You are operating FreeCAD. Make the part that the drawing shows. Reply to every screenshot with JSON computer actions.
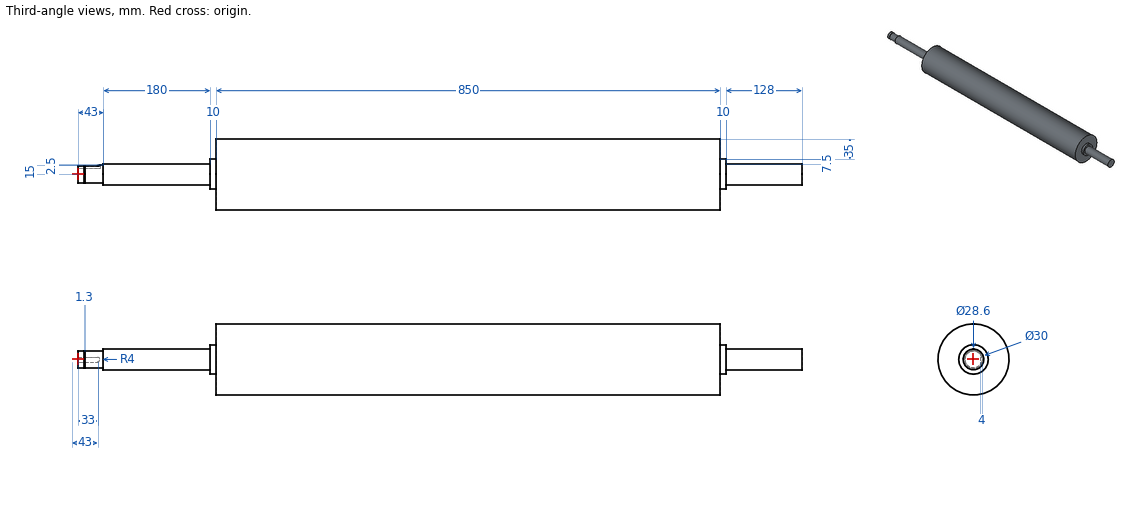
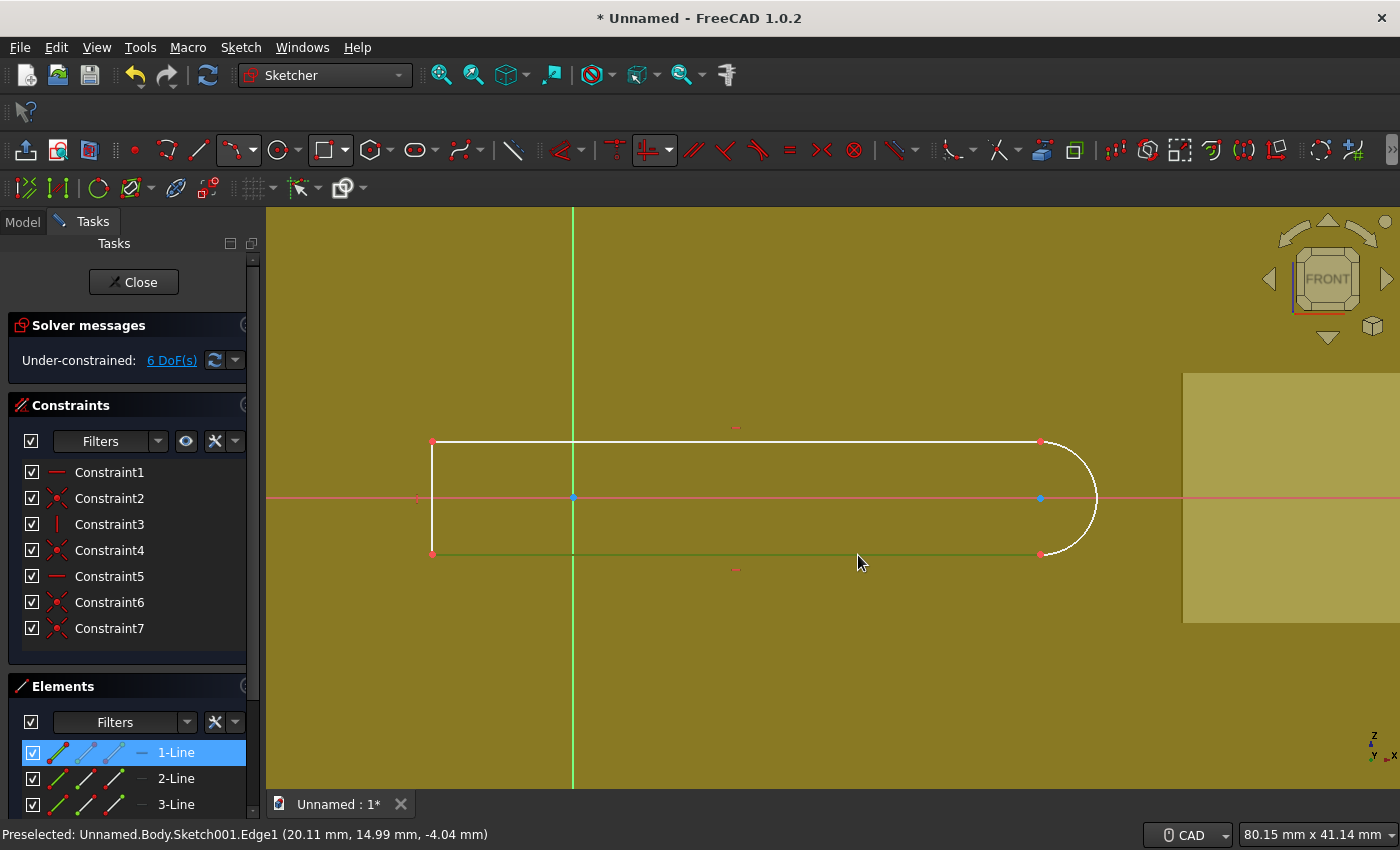
{"action": "left_click", "coordinate": [1086, 532]}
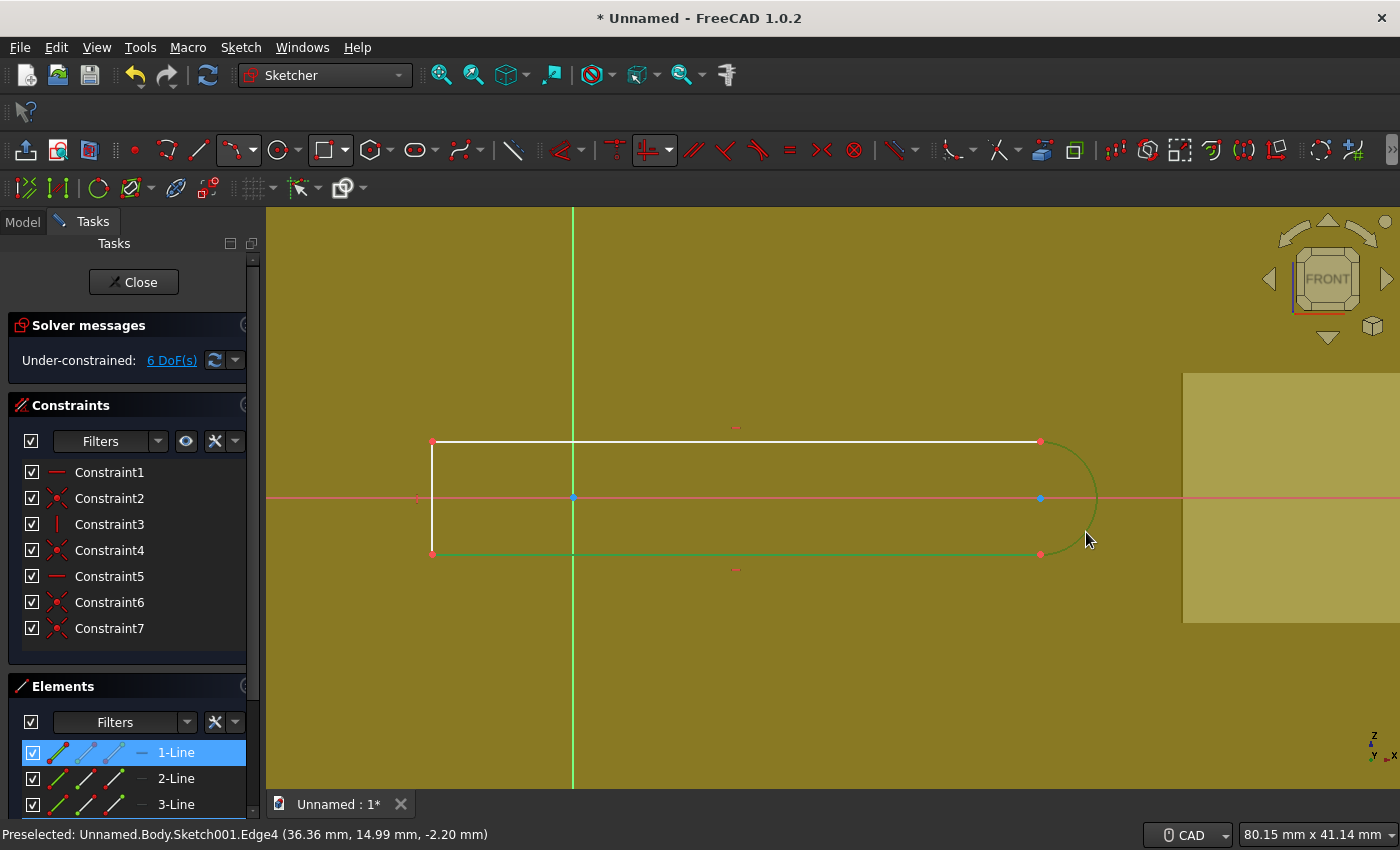
{"action": "key", "text": "t"}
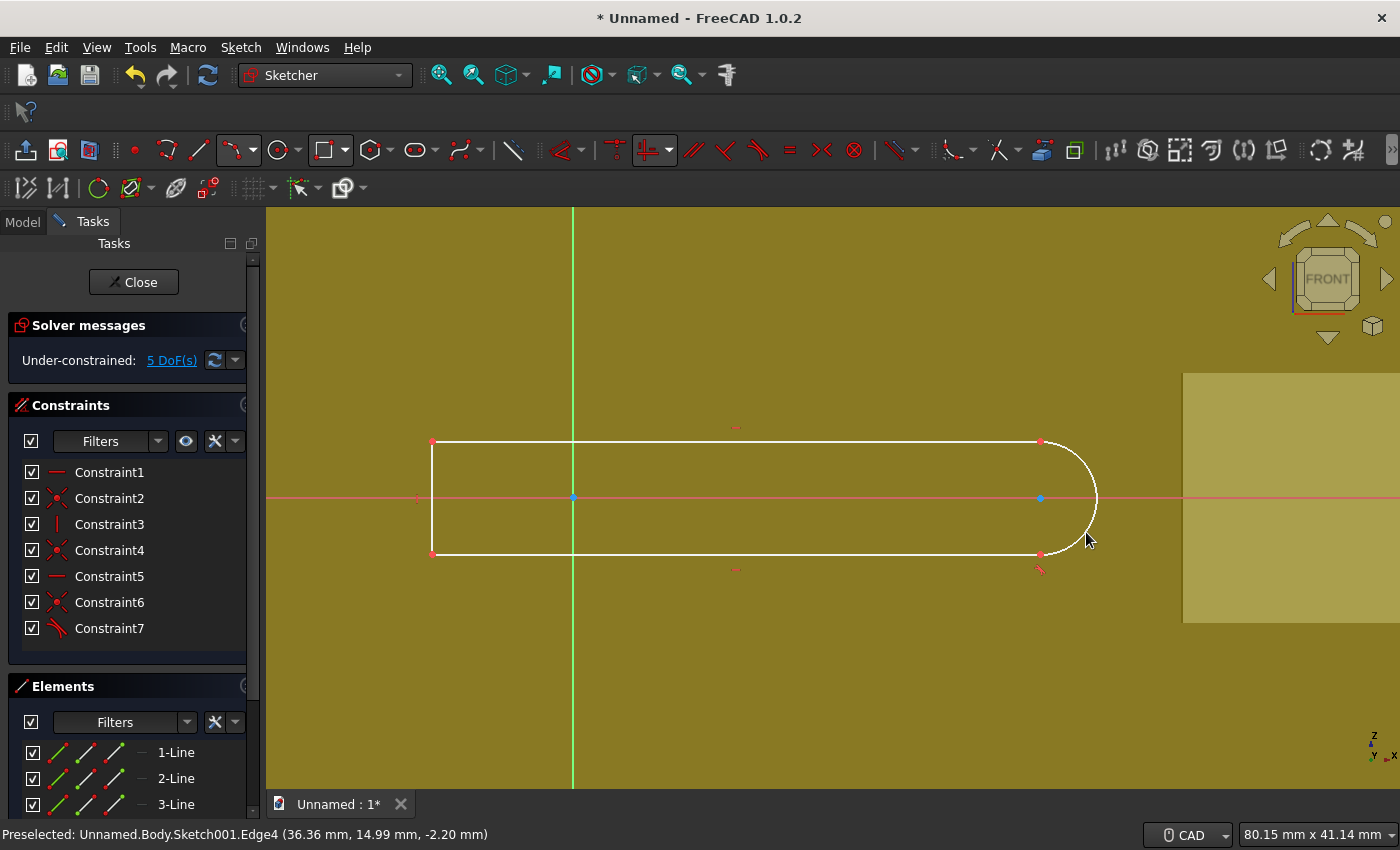
{"action": "left_click", "coordinate": [614, 442]}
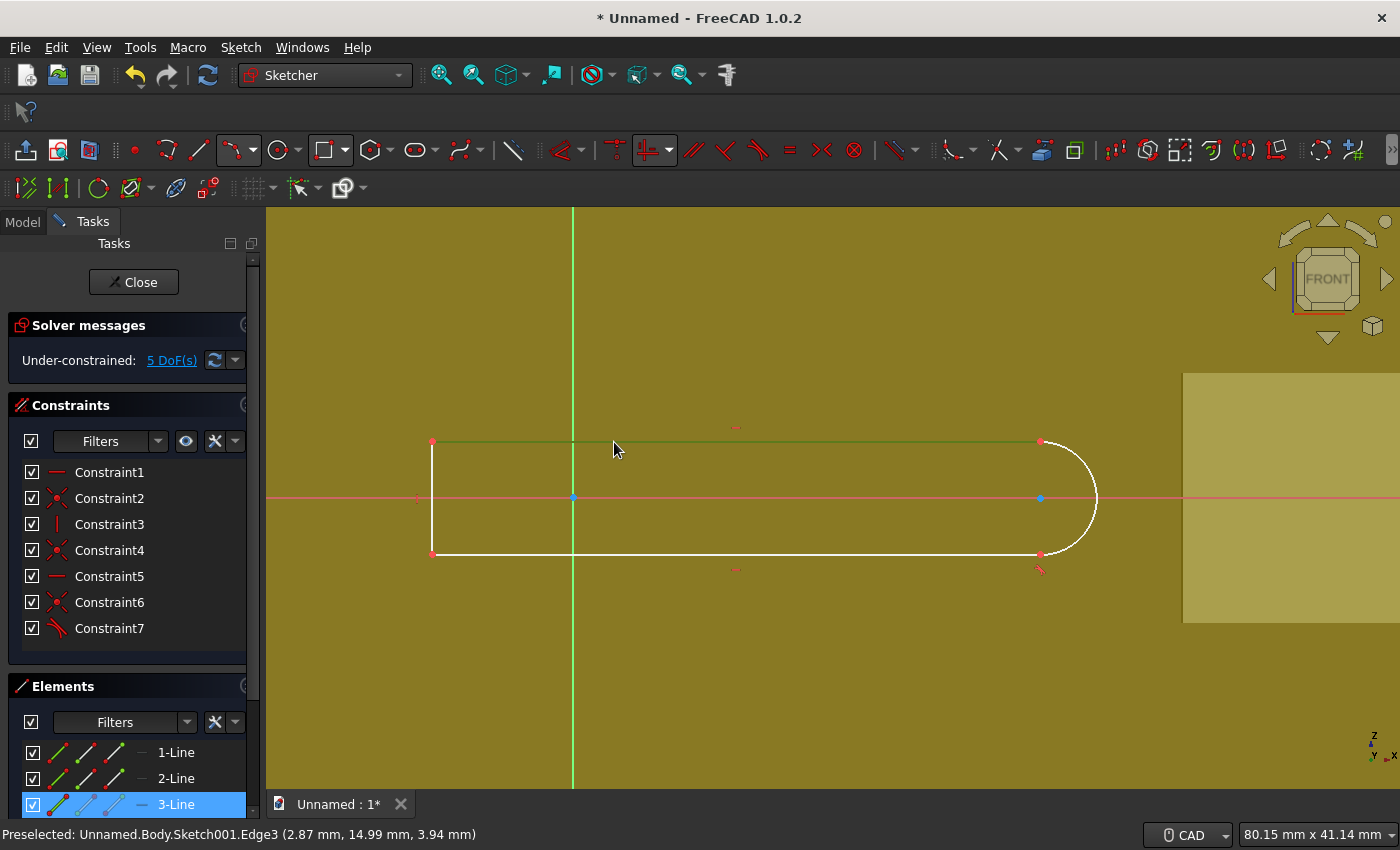
{"action": "left_click", "coordinate": [1086, 532]}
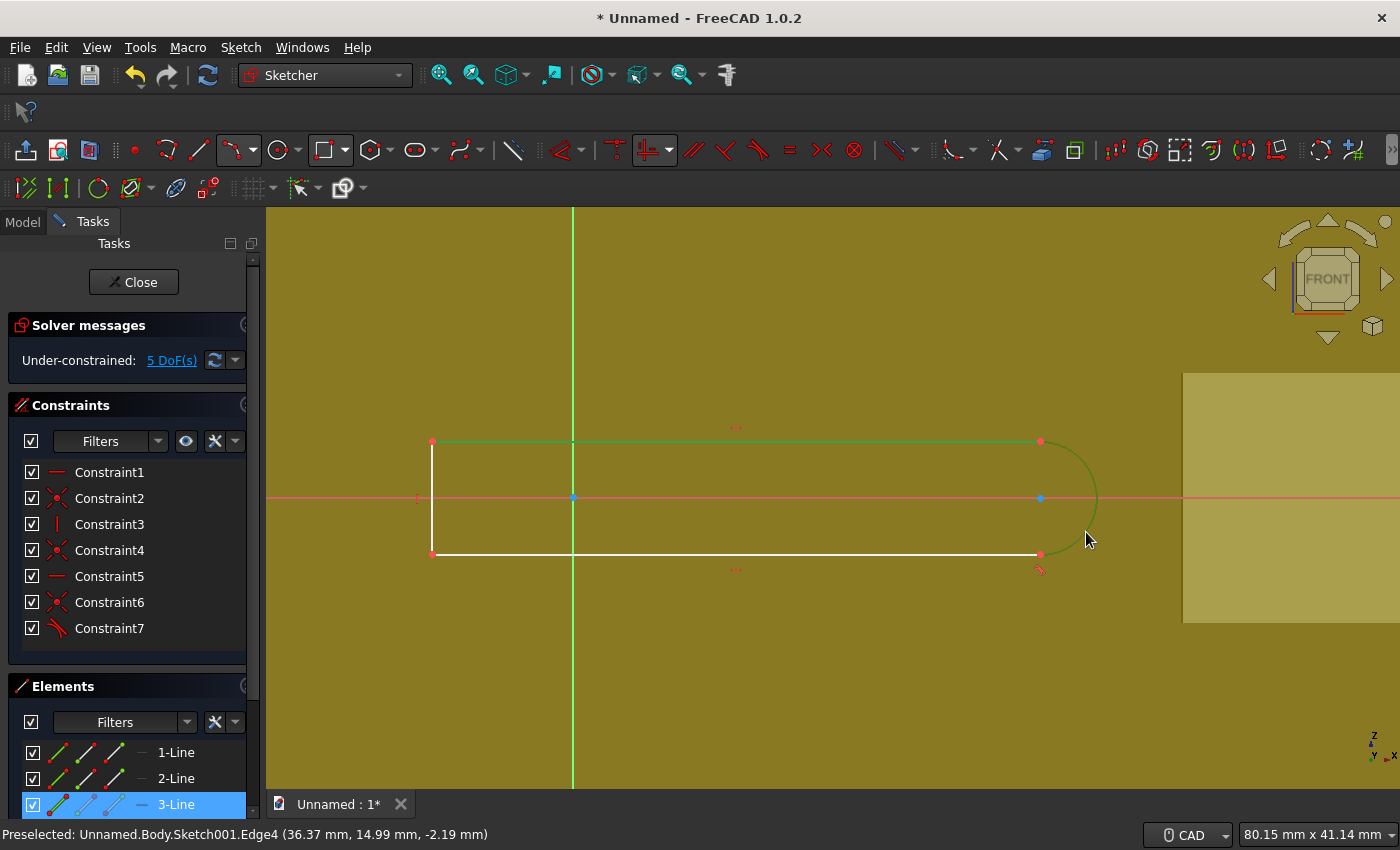
{"action": "left_click", "coordinate": [758, 150]}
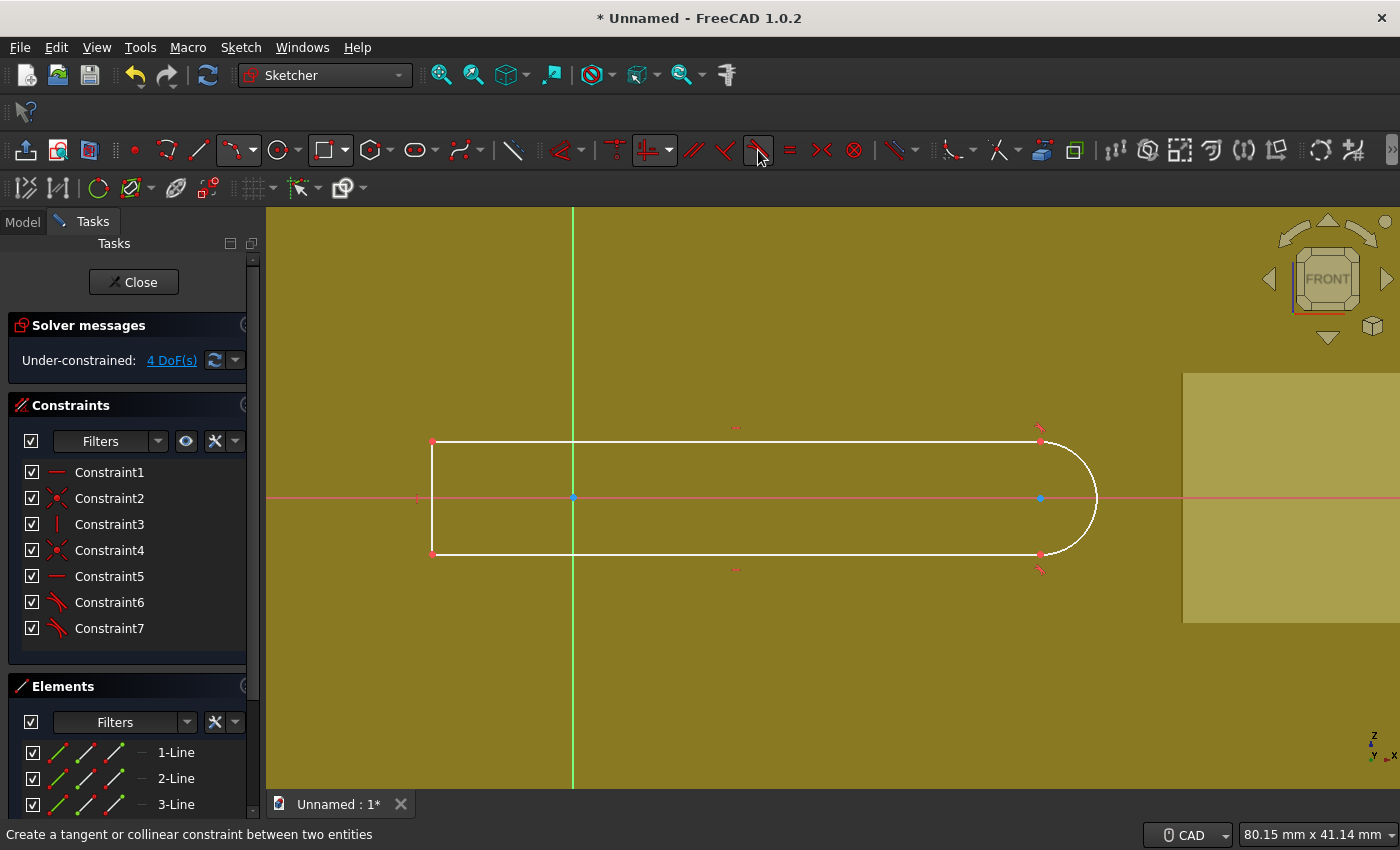
{"action": "left_click", "coordinate": [1040, 498]}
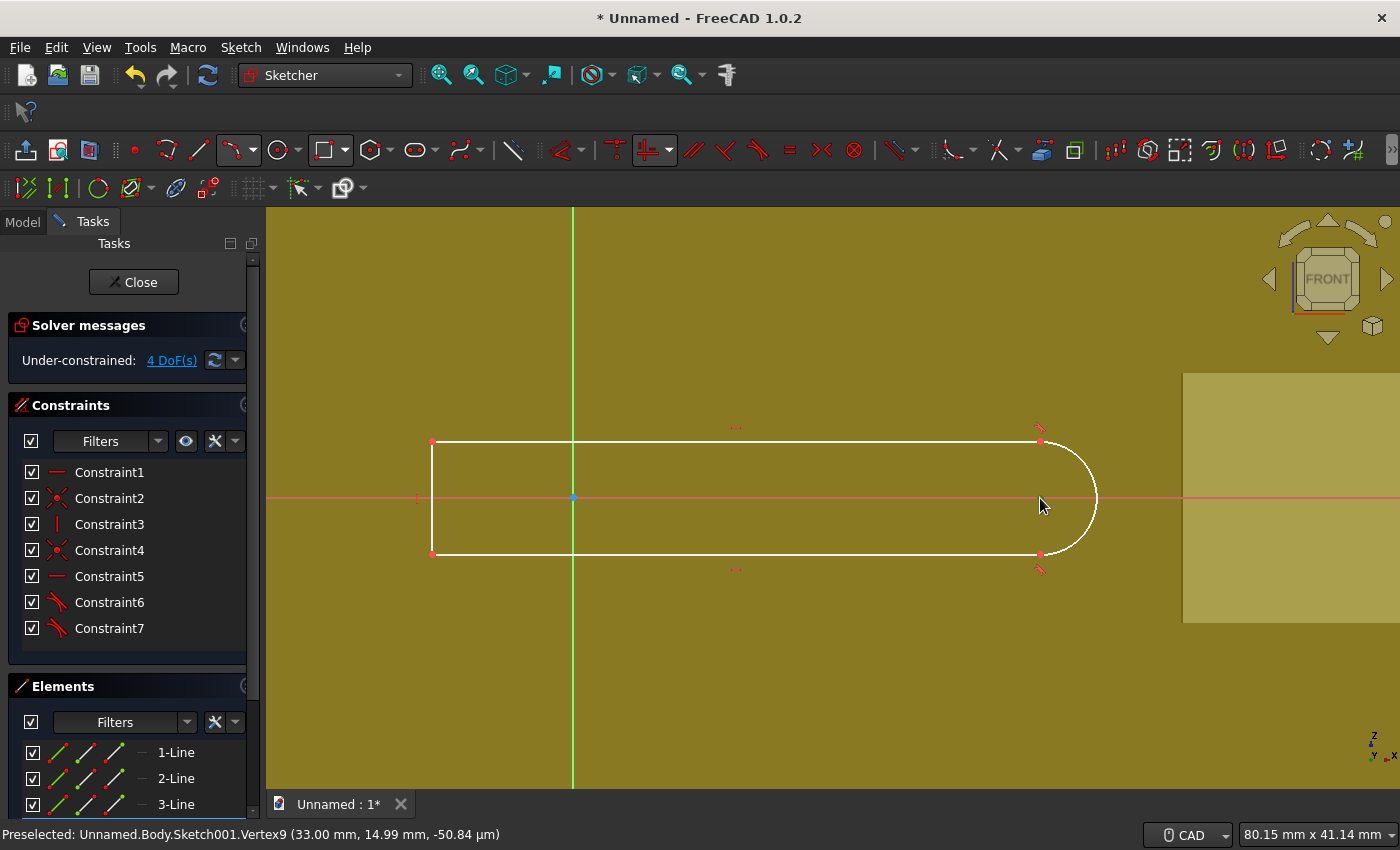
{"action": "left_click", "coordinate": [361, 498]}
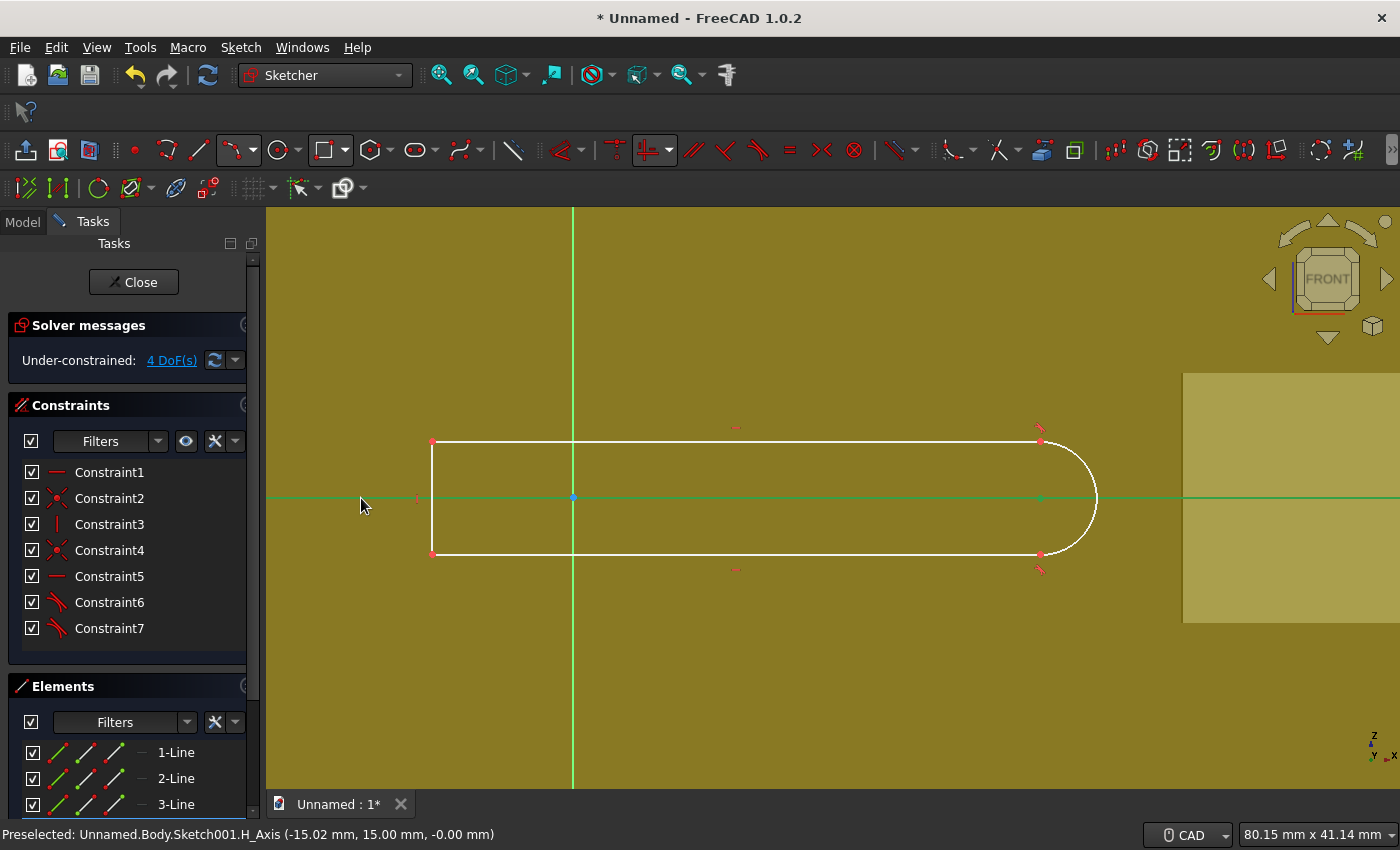
{"action": "key", "text": "c"}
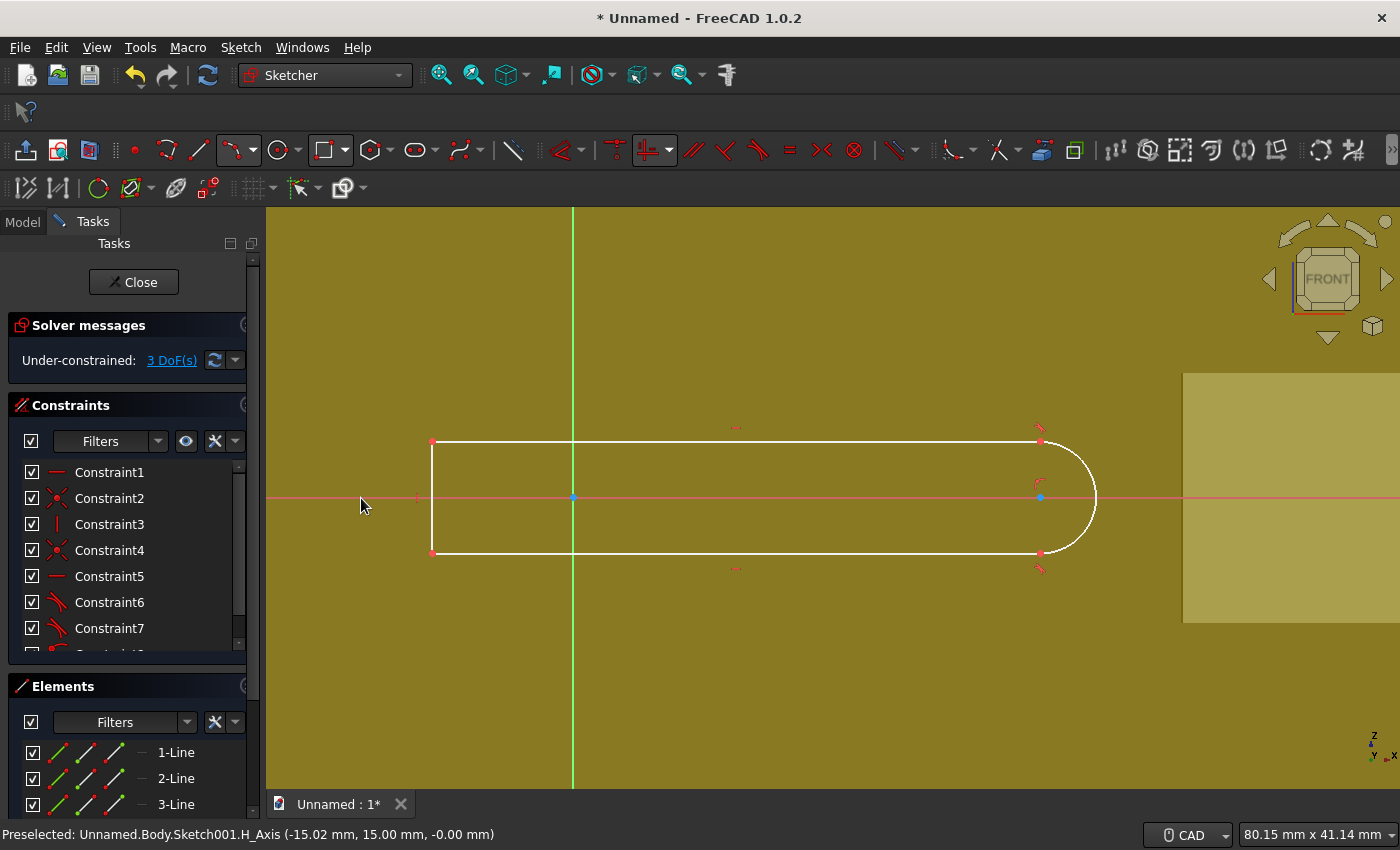
{"action": "left_click", "coordinate": [560, 150]}